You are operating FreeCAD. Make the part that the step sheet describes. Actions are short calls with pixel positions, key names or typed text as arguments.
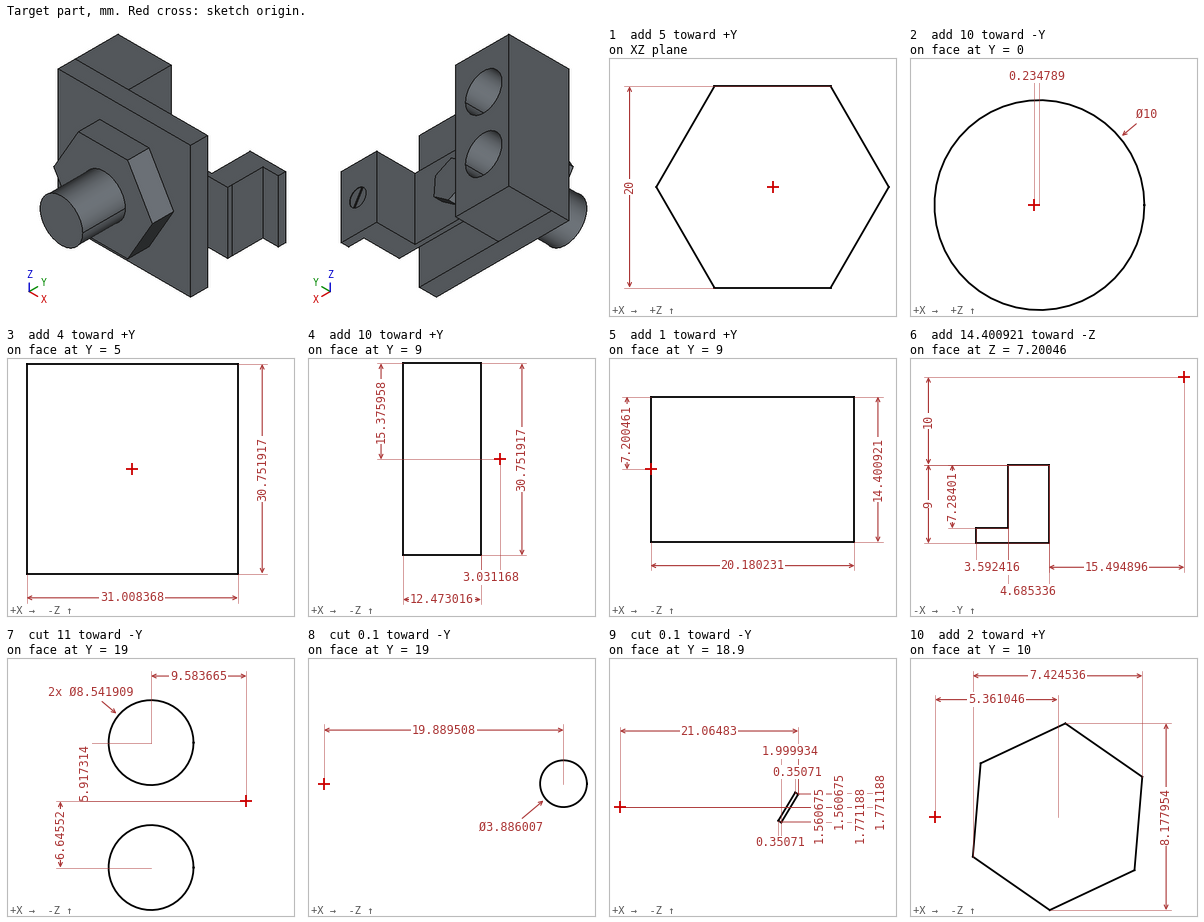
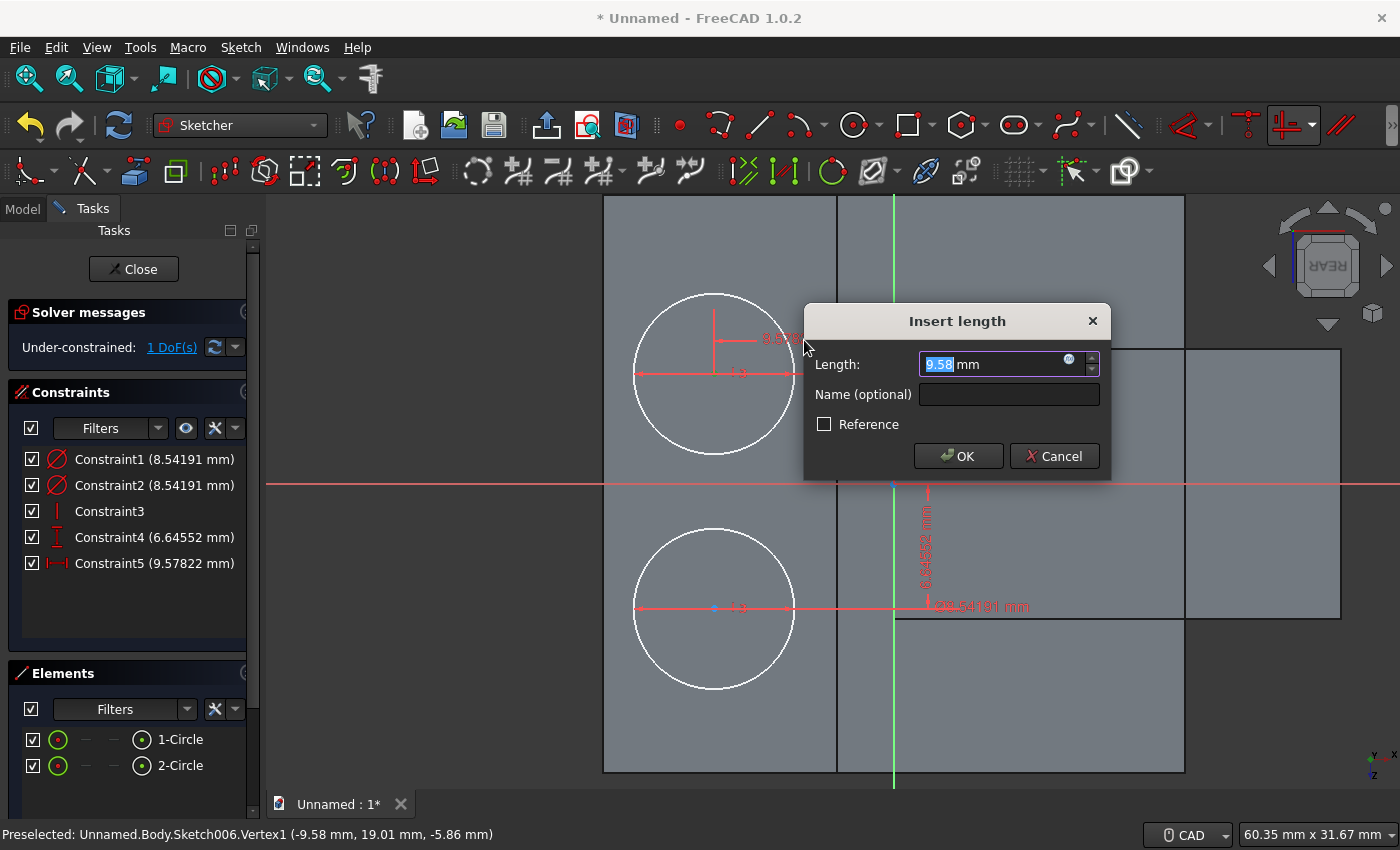
text(9.583665)
key(Return)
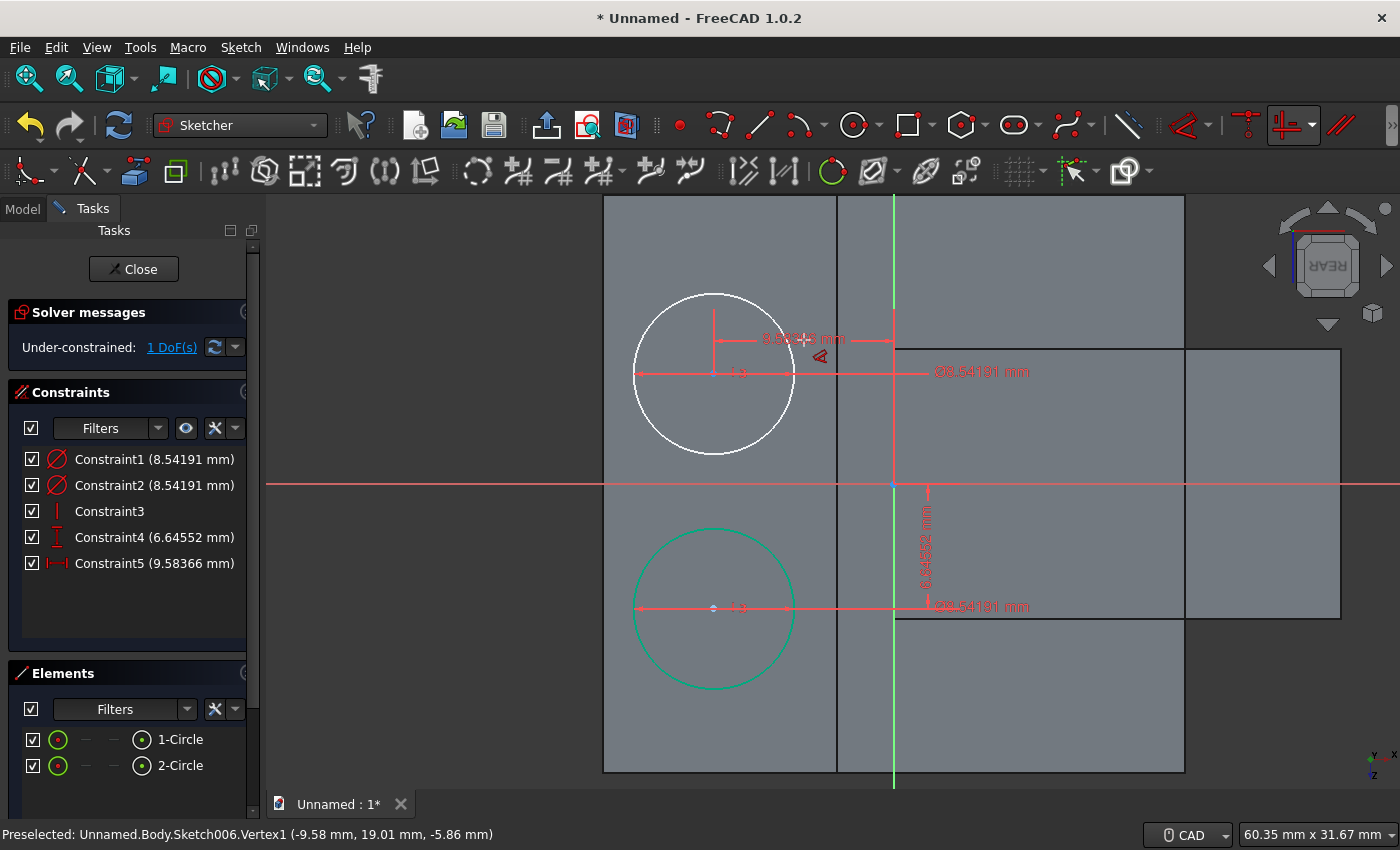
click(714, 374)
click(928, 429)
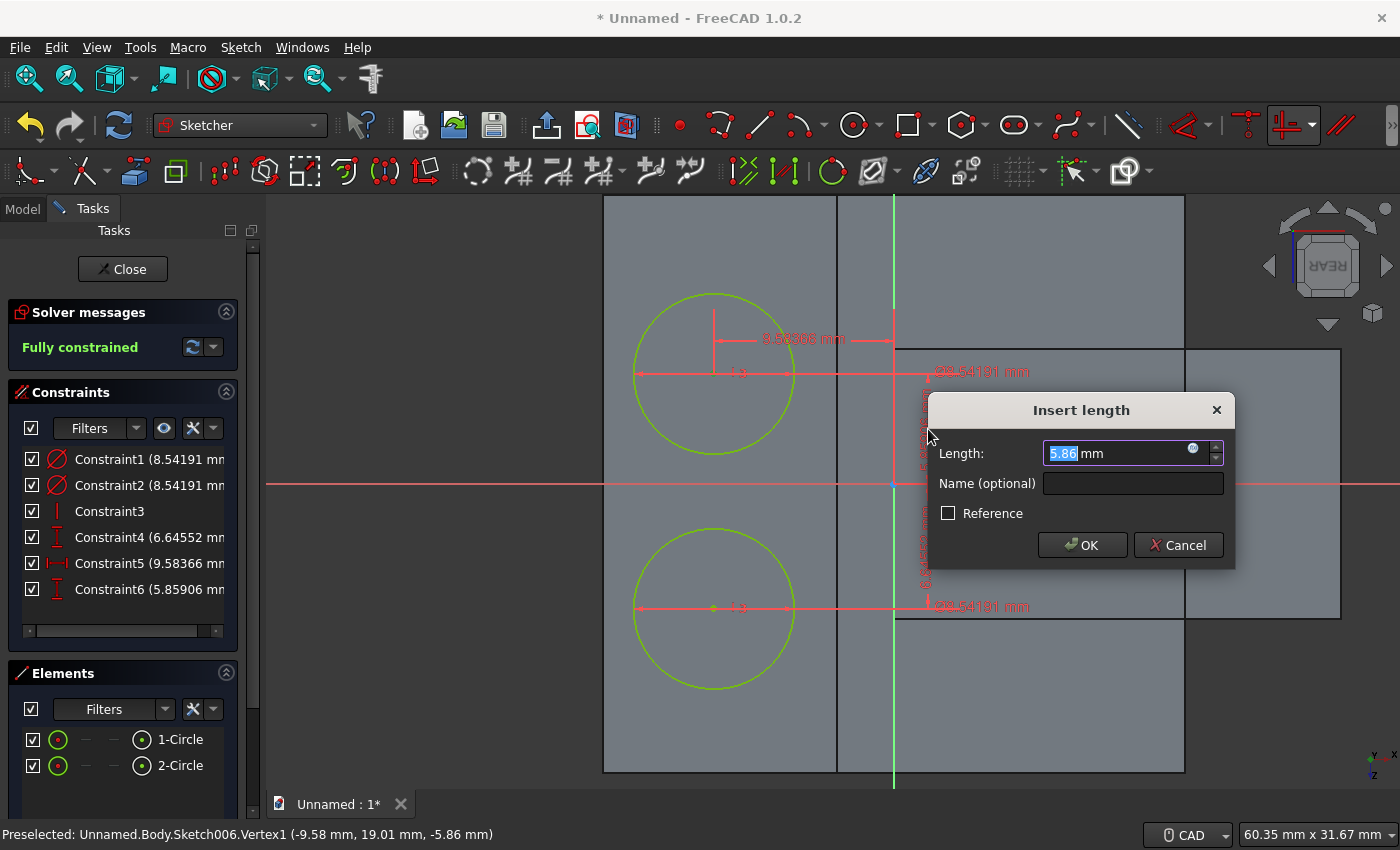
text(5.917314)
key(Return)
key(Escape)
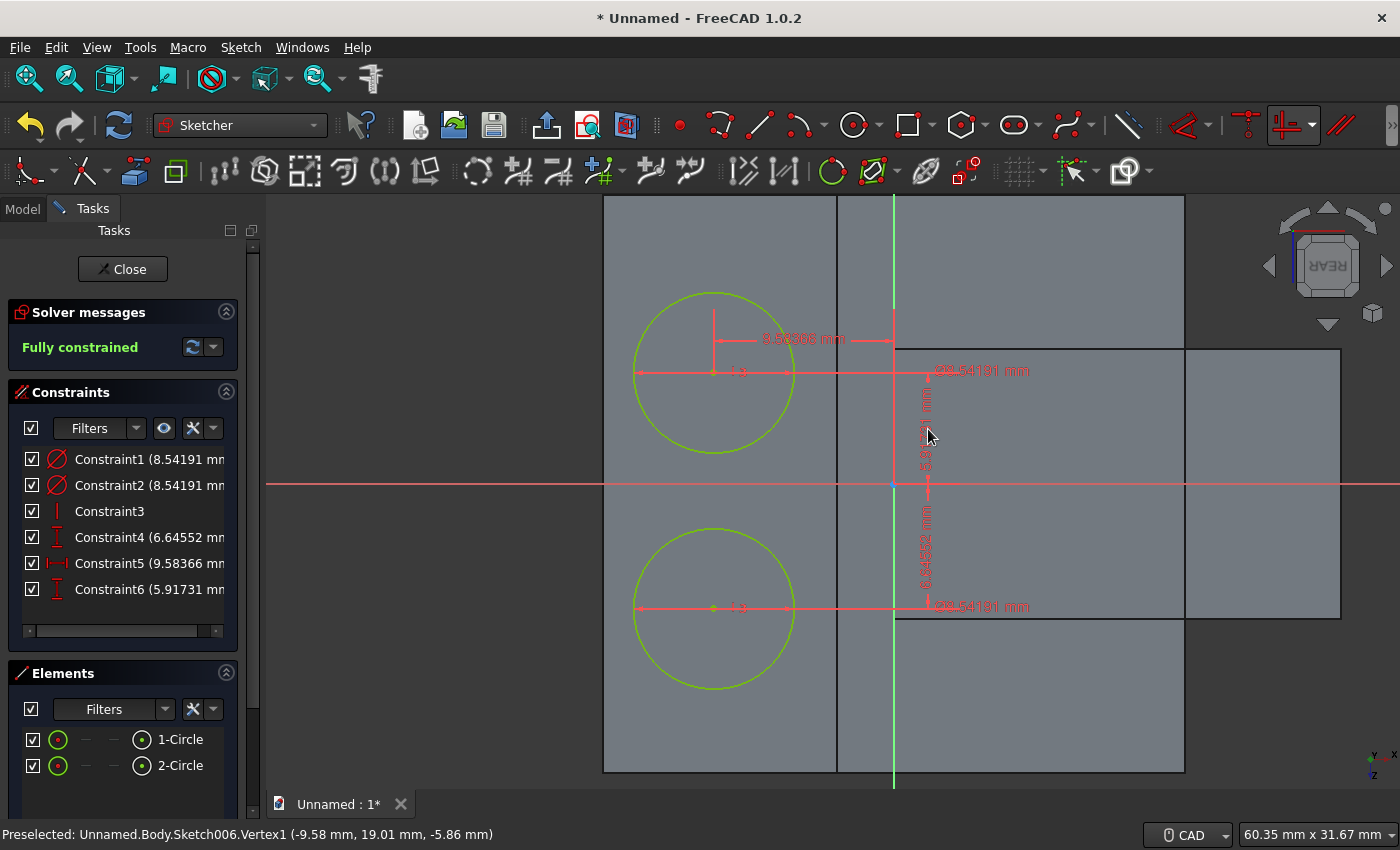
click(123, 269)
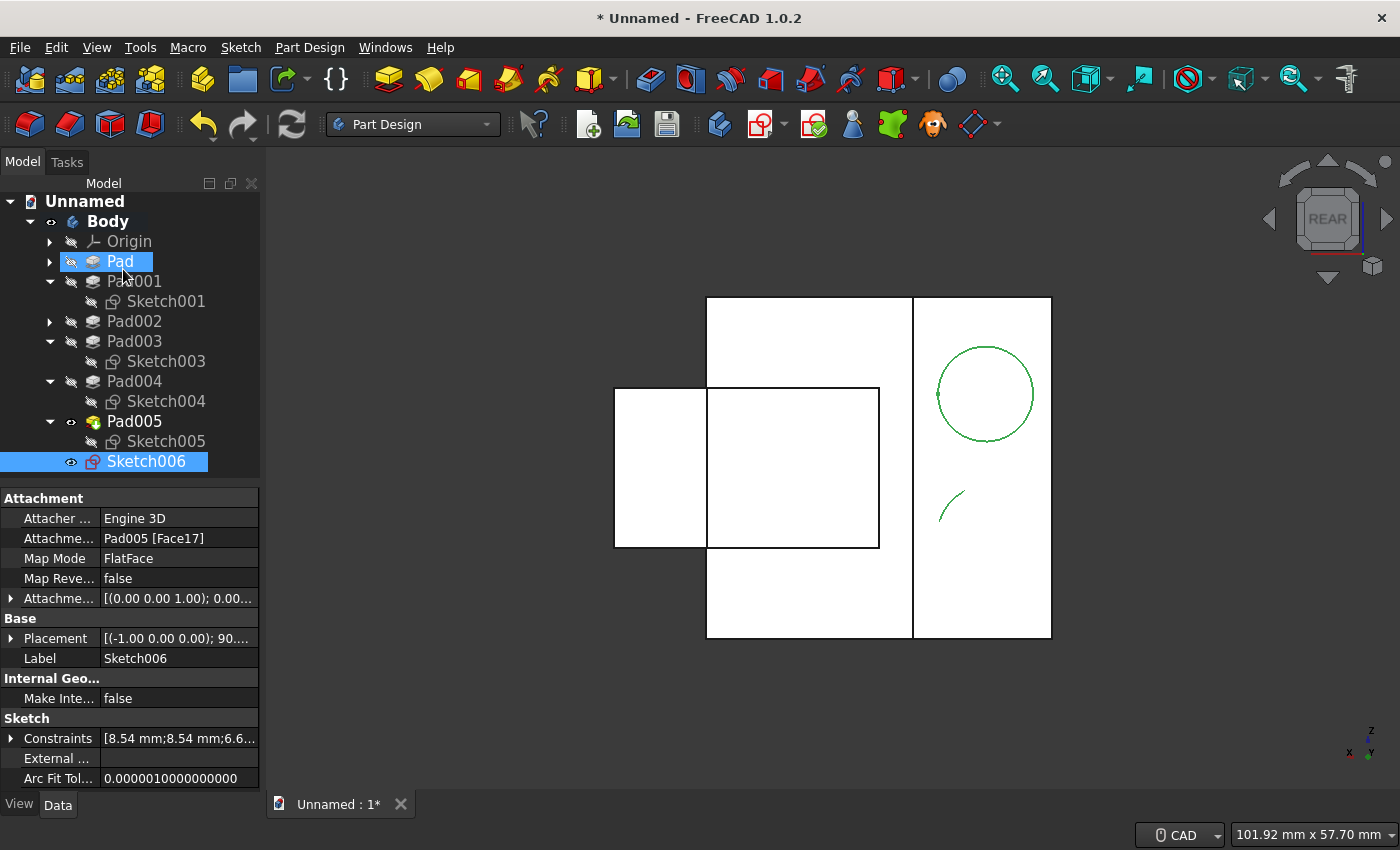
click(652, 80)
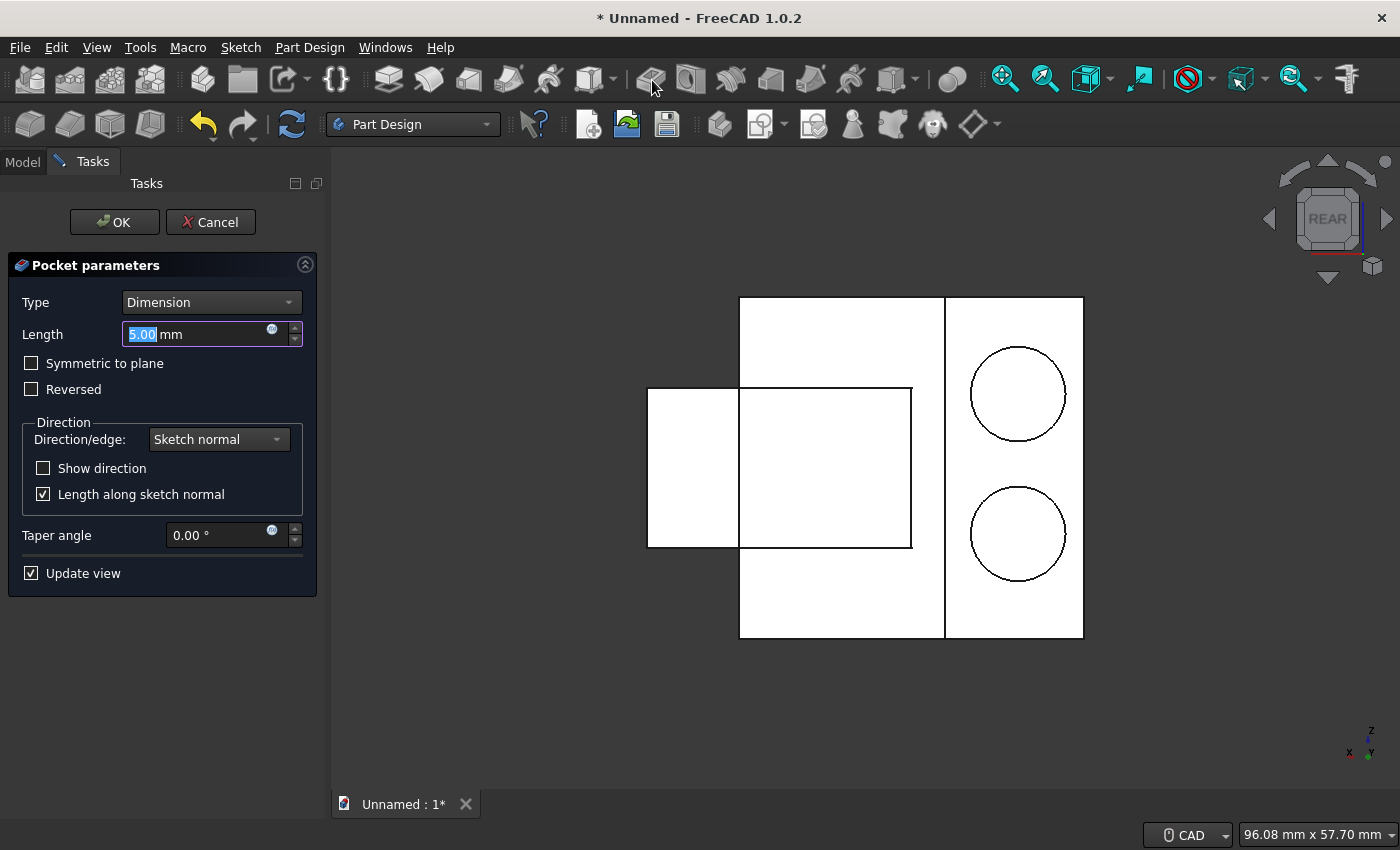
text(11)
key(Tab)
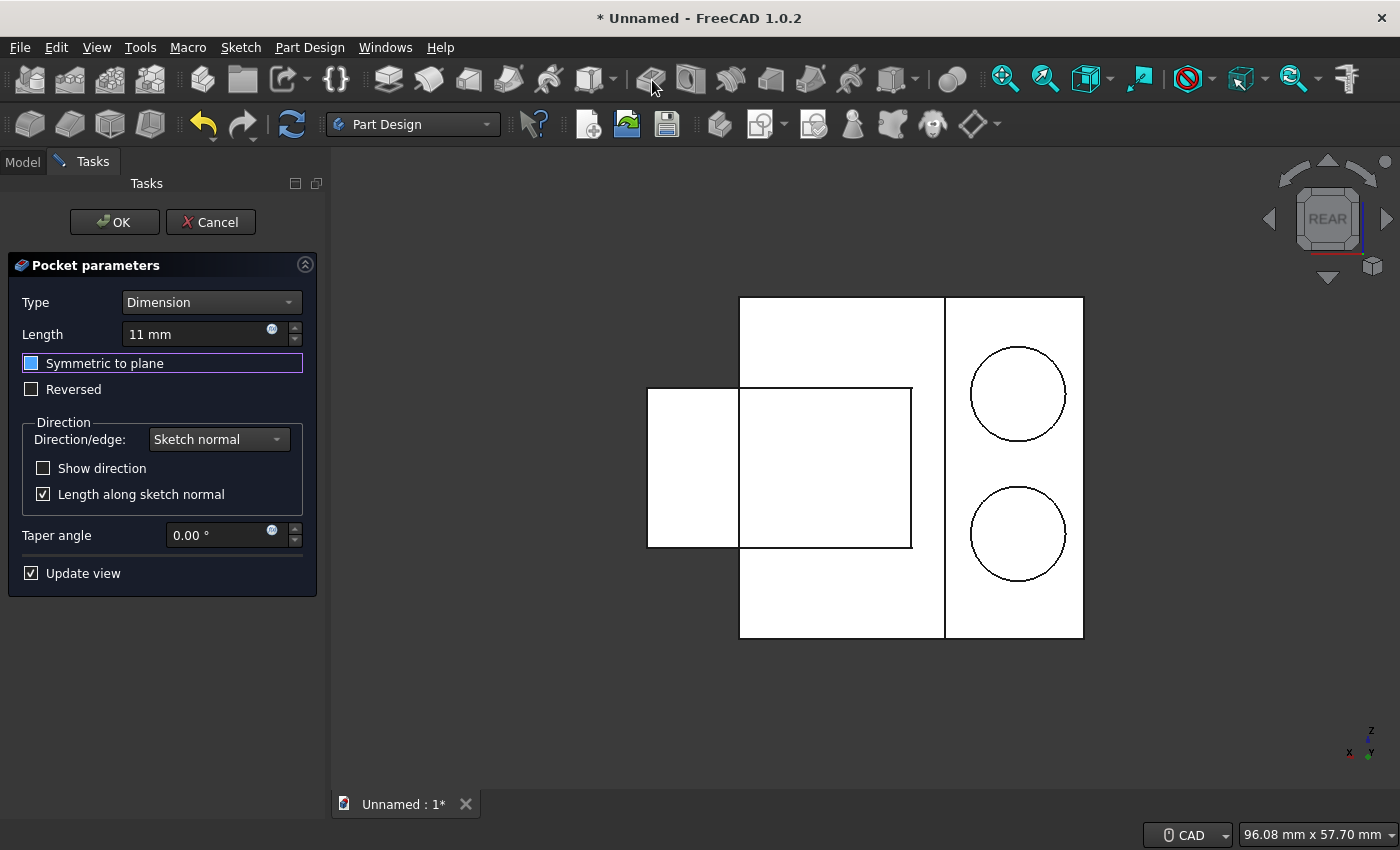
click(115, 222)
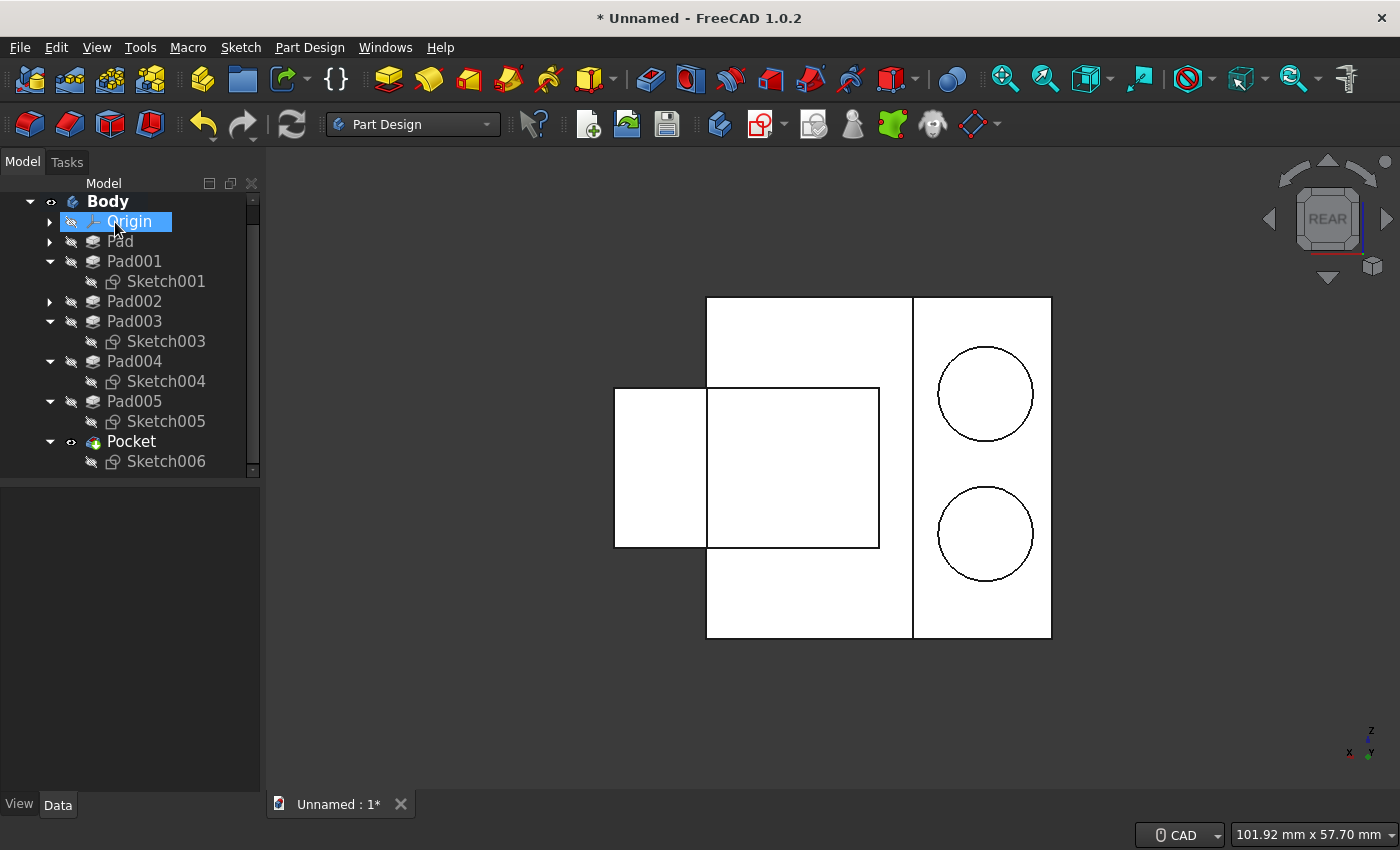
click(942, 467)